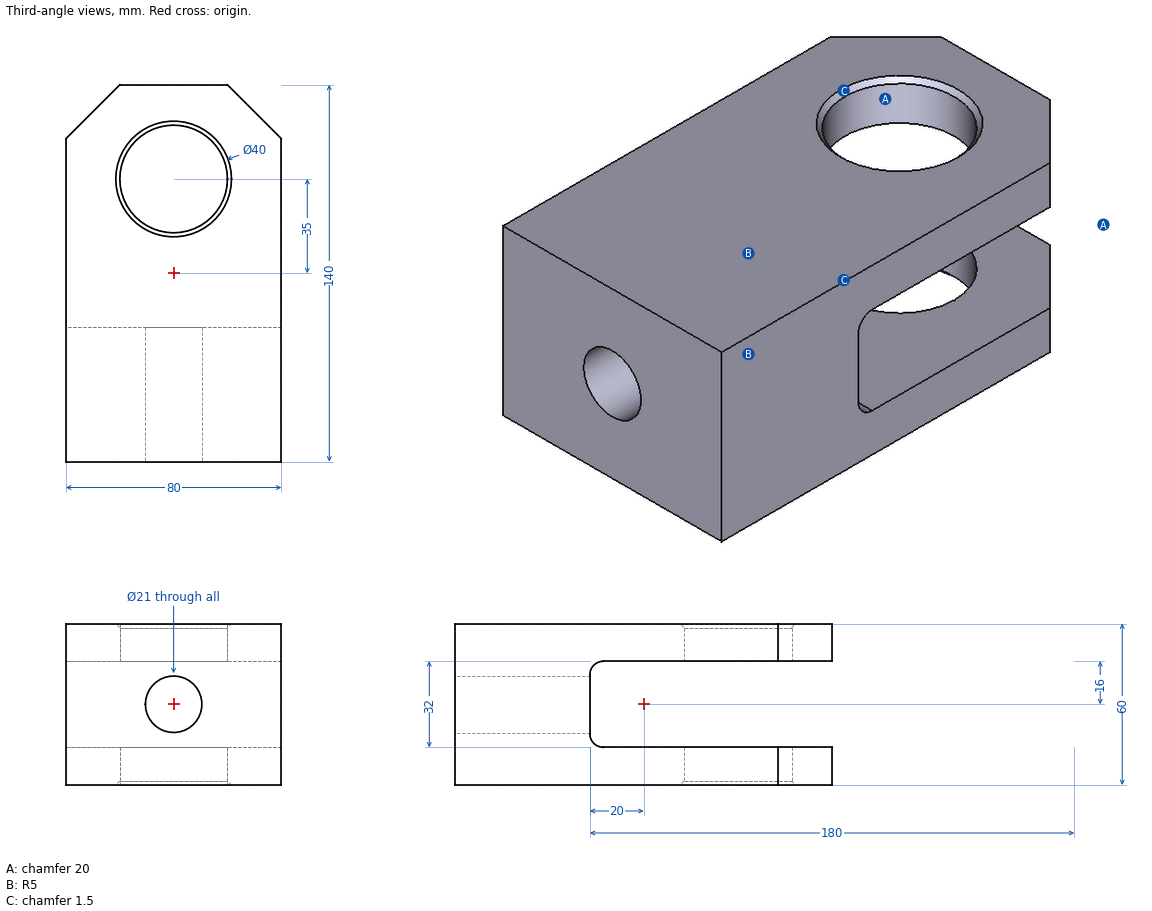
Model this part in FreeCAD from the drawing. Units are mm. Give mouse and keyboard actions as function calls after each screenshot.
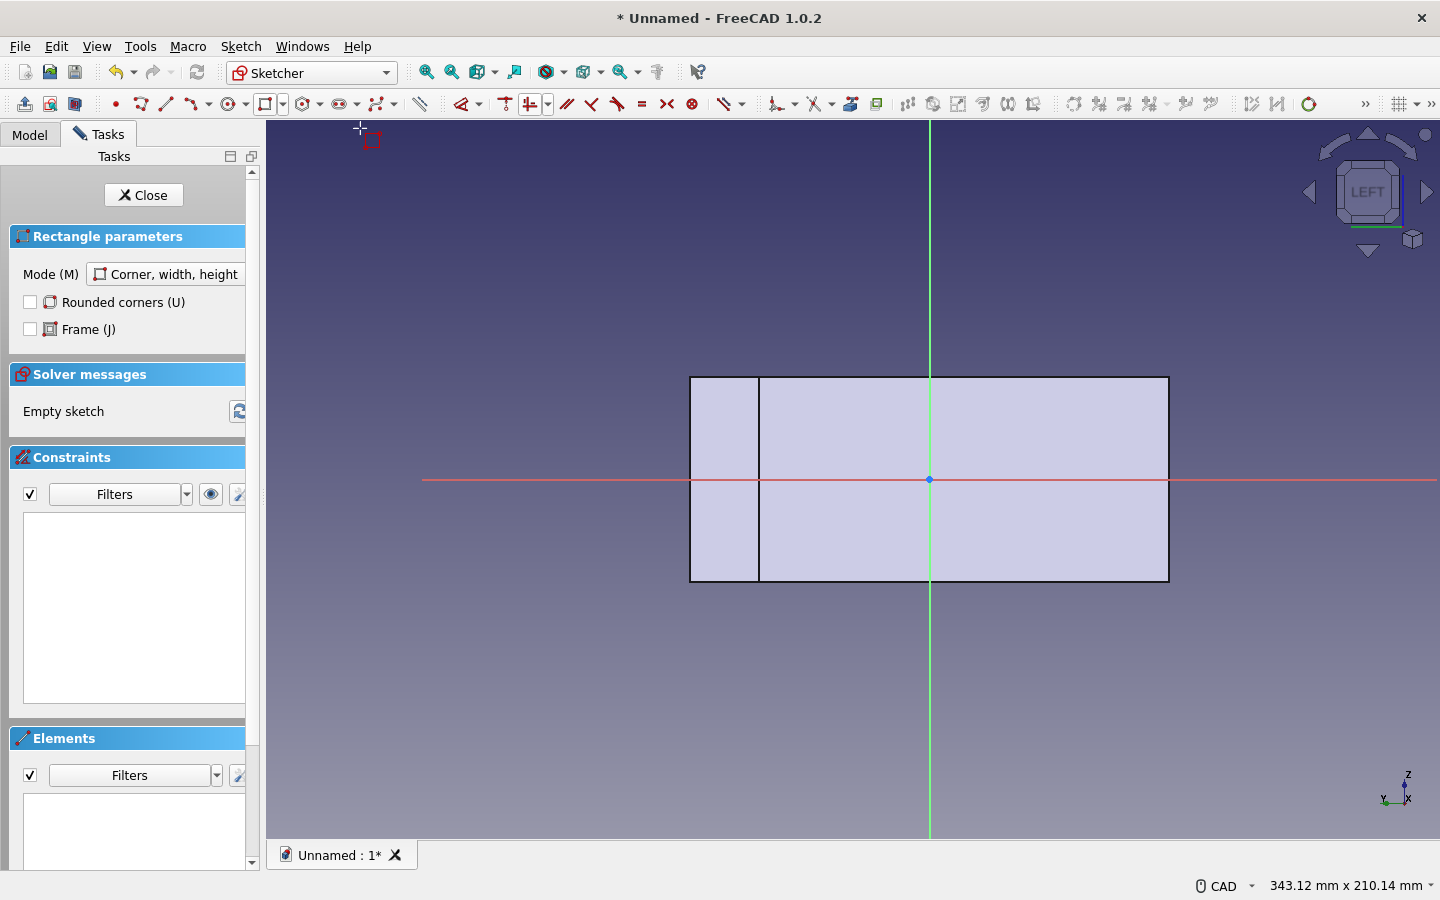
click(382, 425)
move(998, 534)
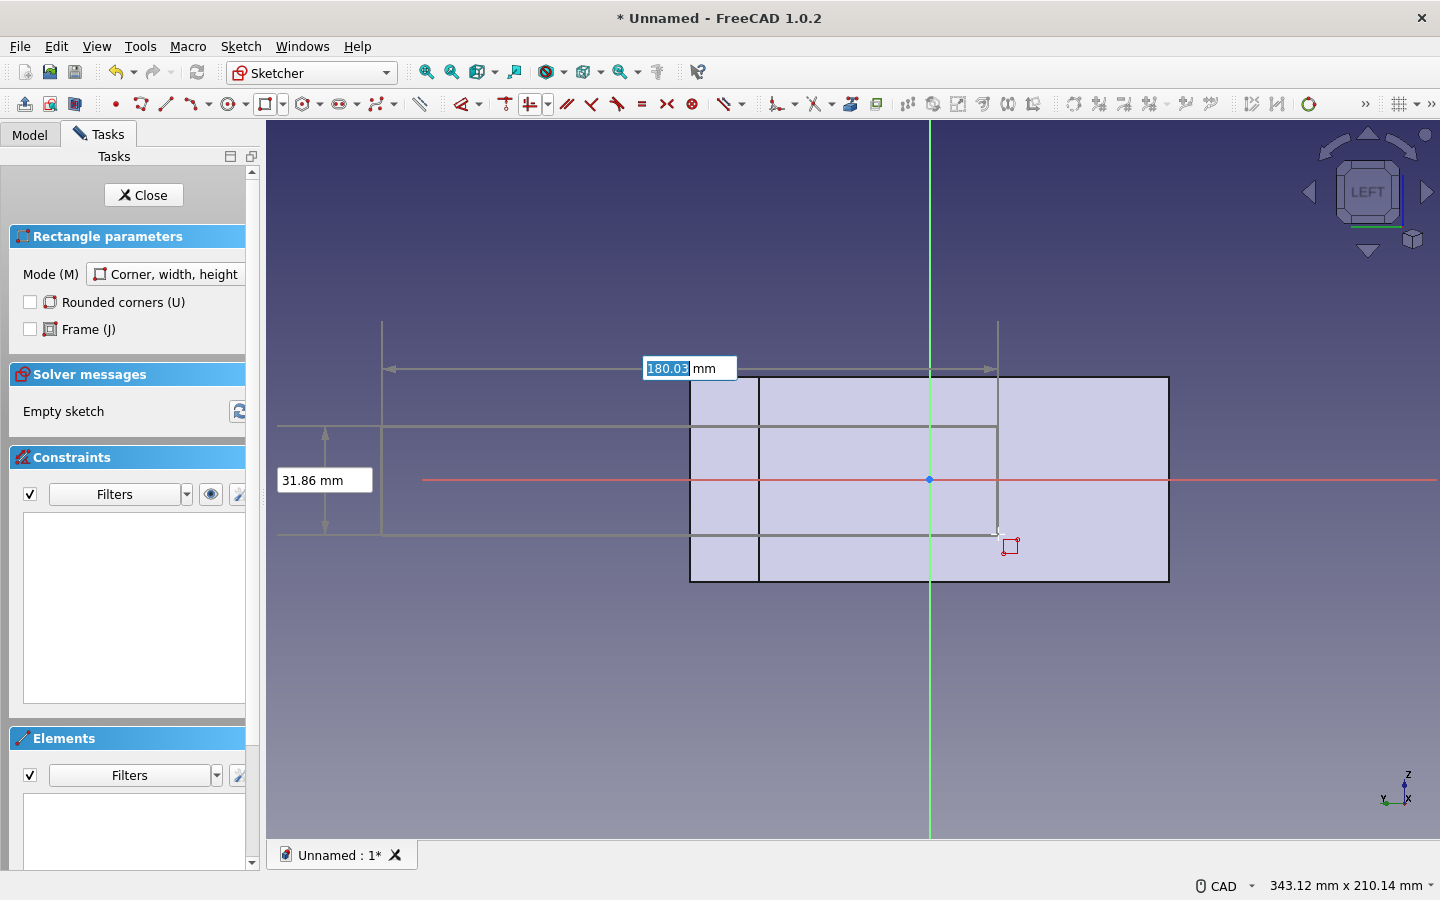
text(180)
key(Tab)
text(32)
key(Return)
key(Escape)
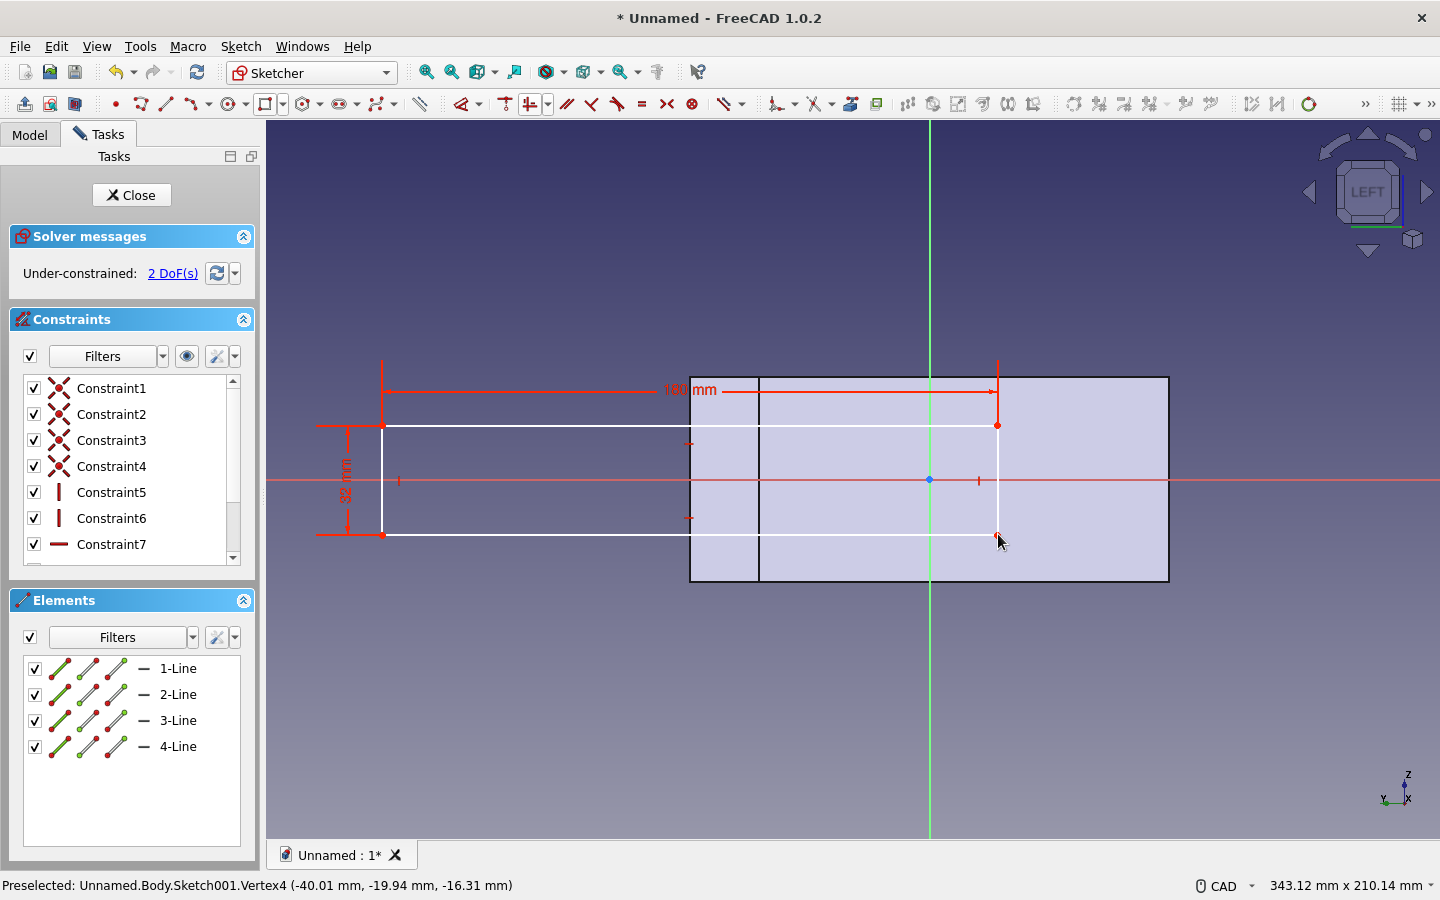
click(460, 104)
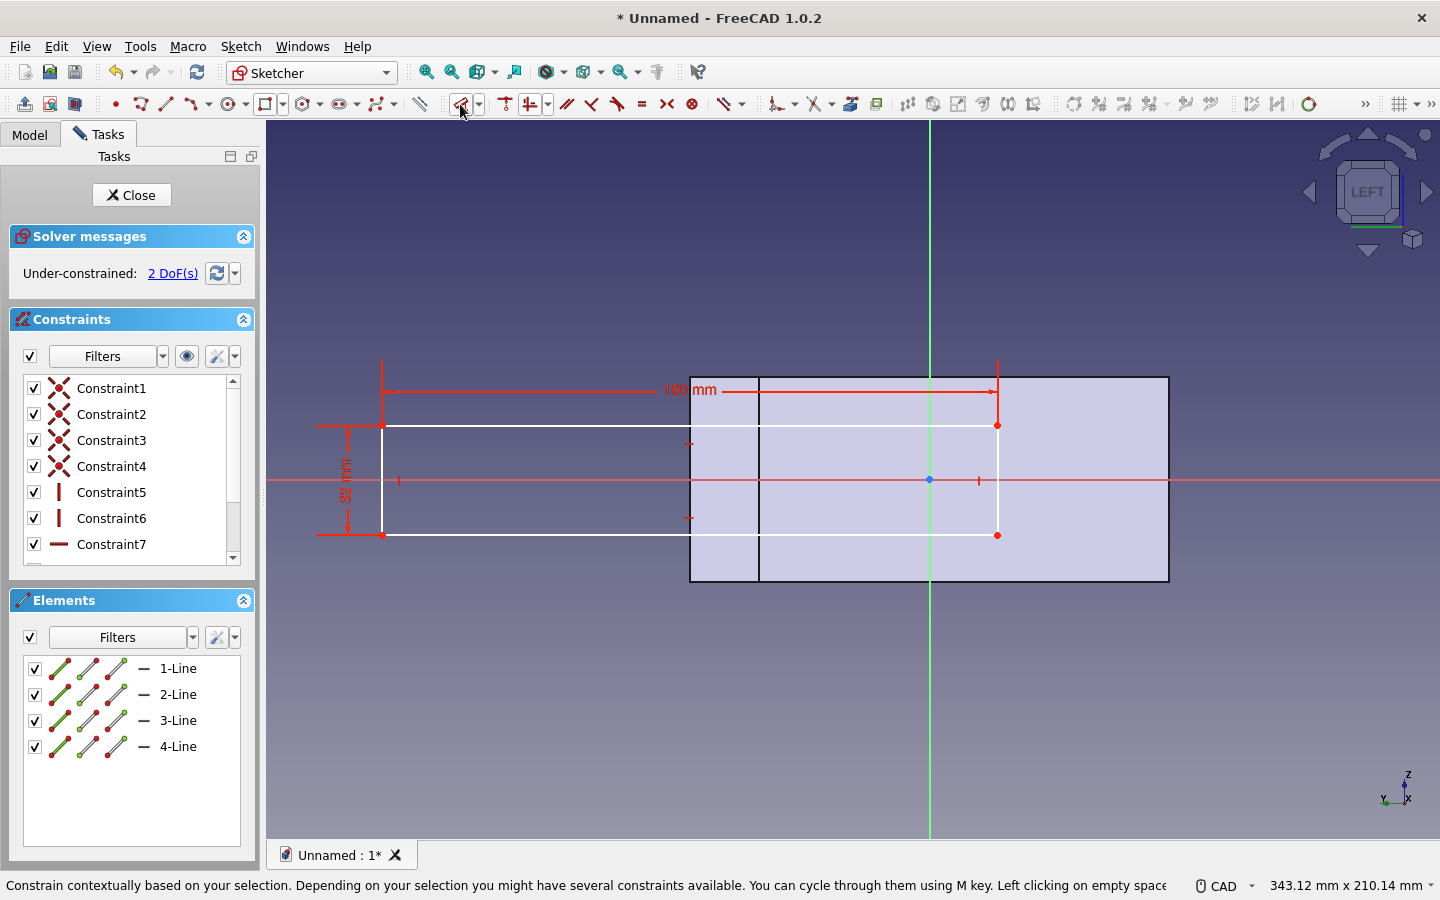
click(382, 426)
click(348, 453)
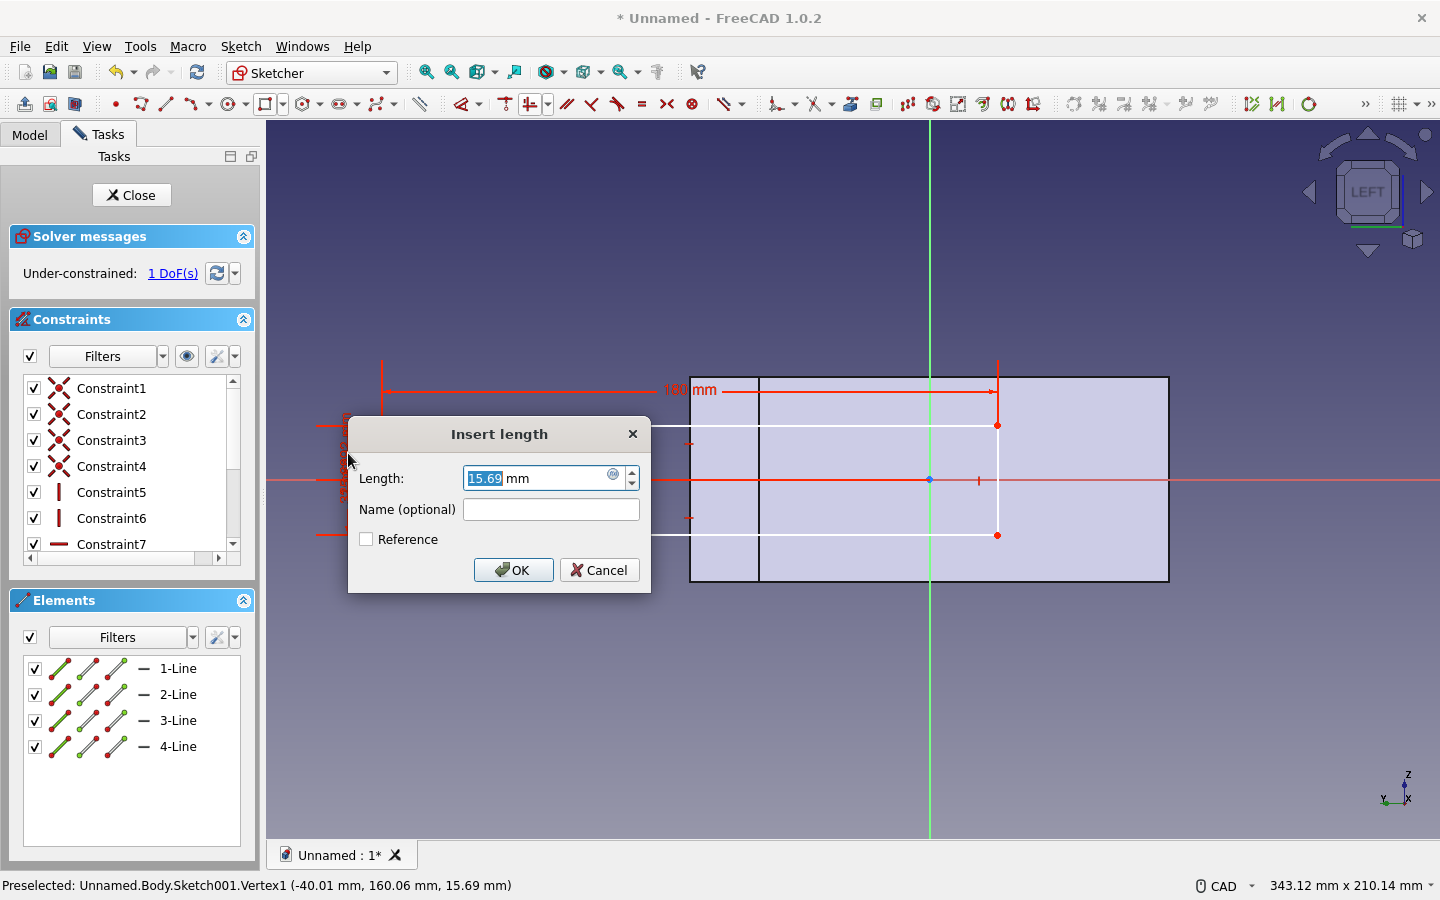
text(16)
key(Return)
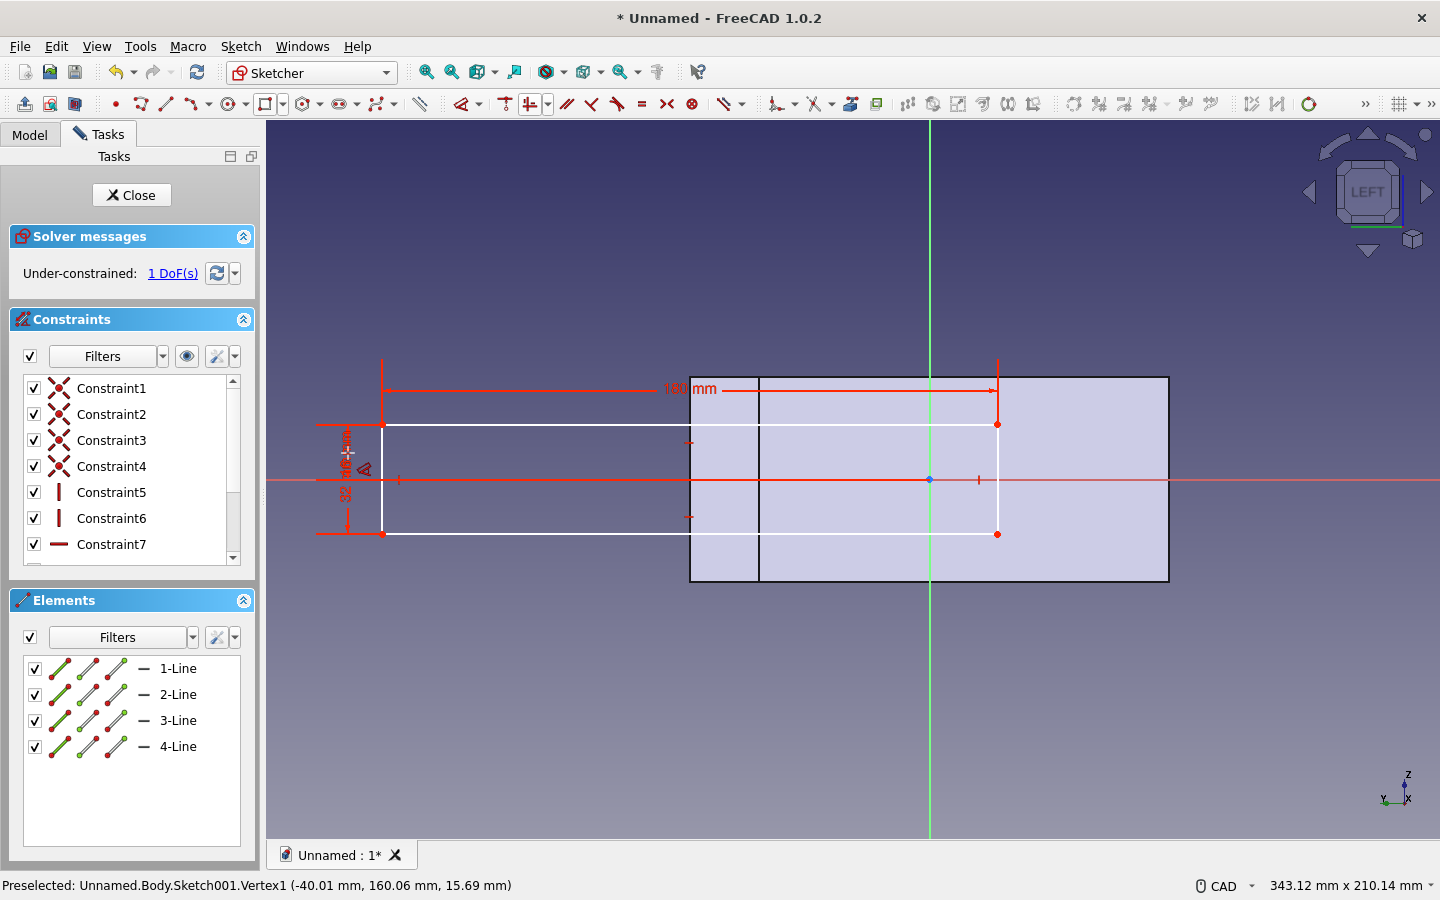
click(998, 534)
click(964, 568)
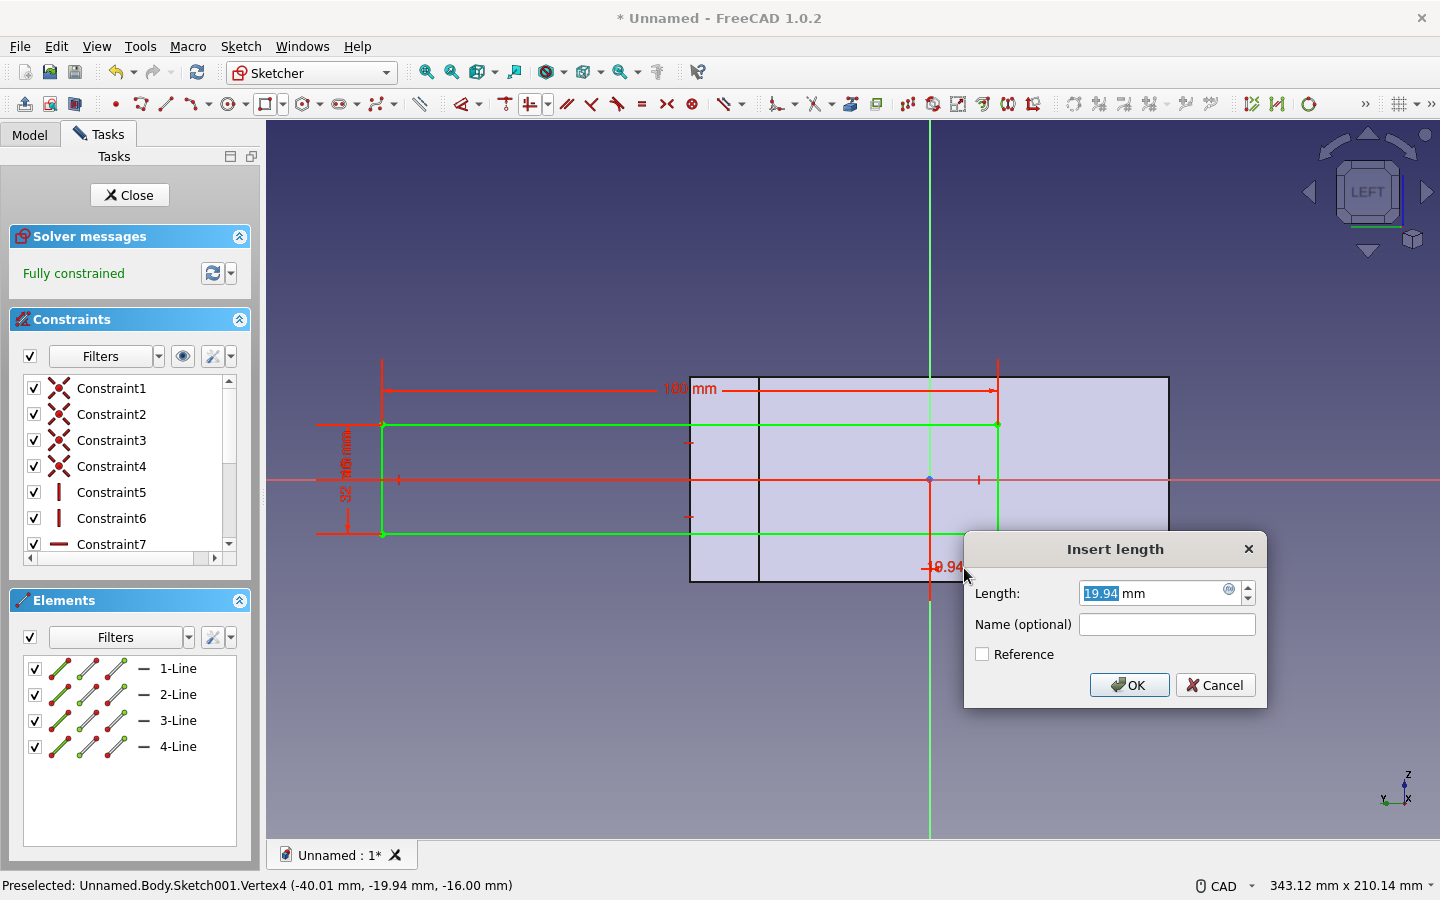
text(20)
key(Return)
key(Escape)